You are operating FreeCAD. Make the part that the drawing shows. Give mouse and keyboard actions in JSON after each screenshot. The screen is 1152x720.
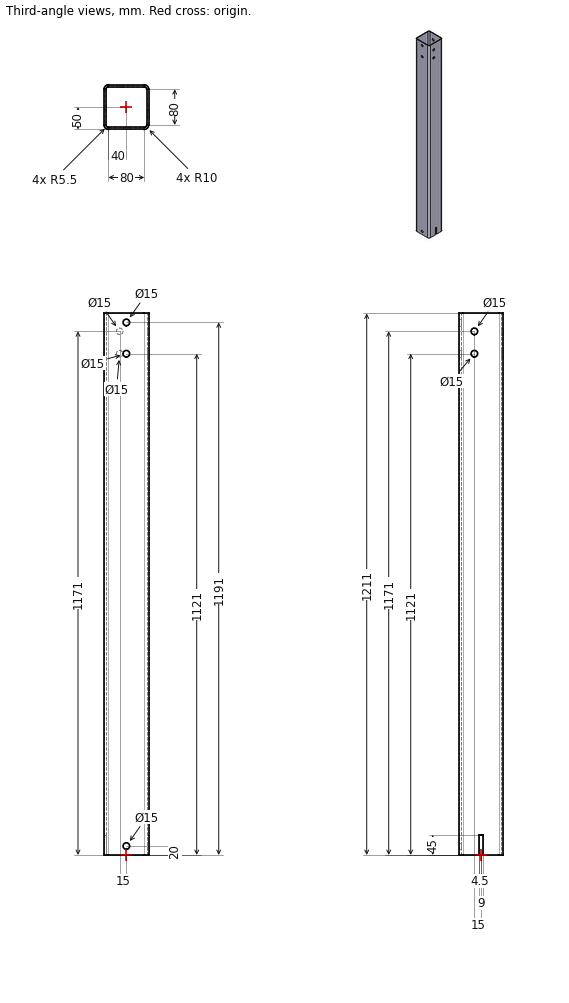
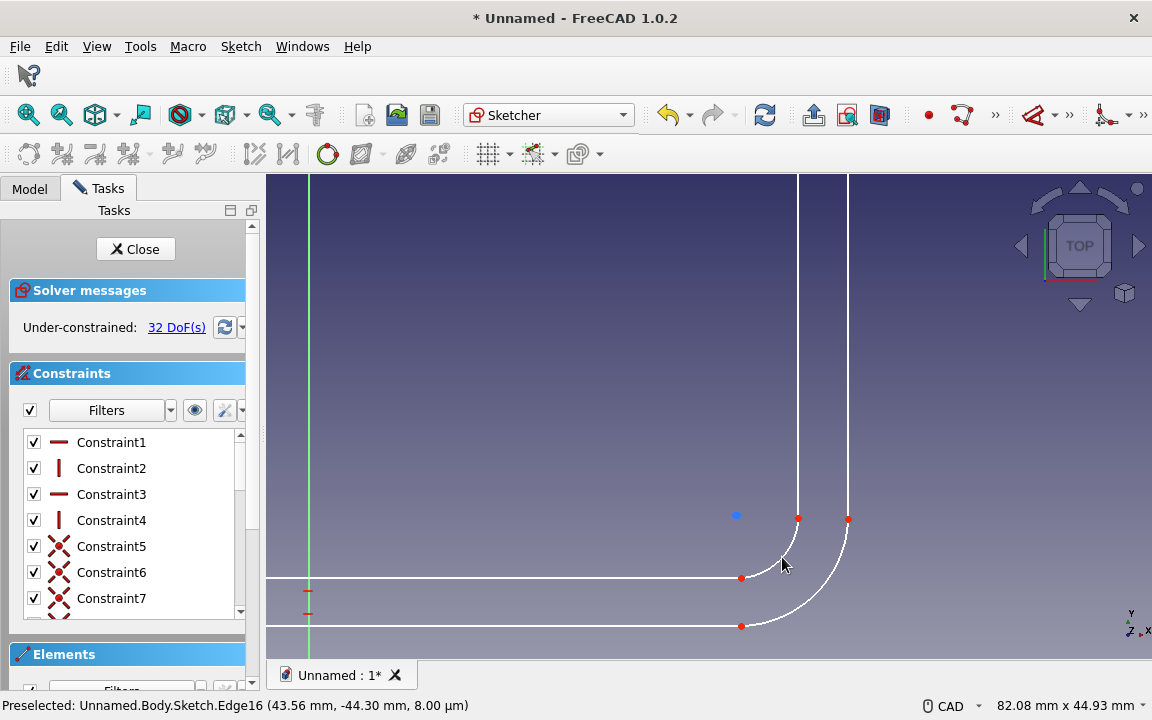
{"action": "left_click", "coordinate": [482, 626]}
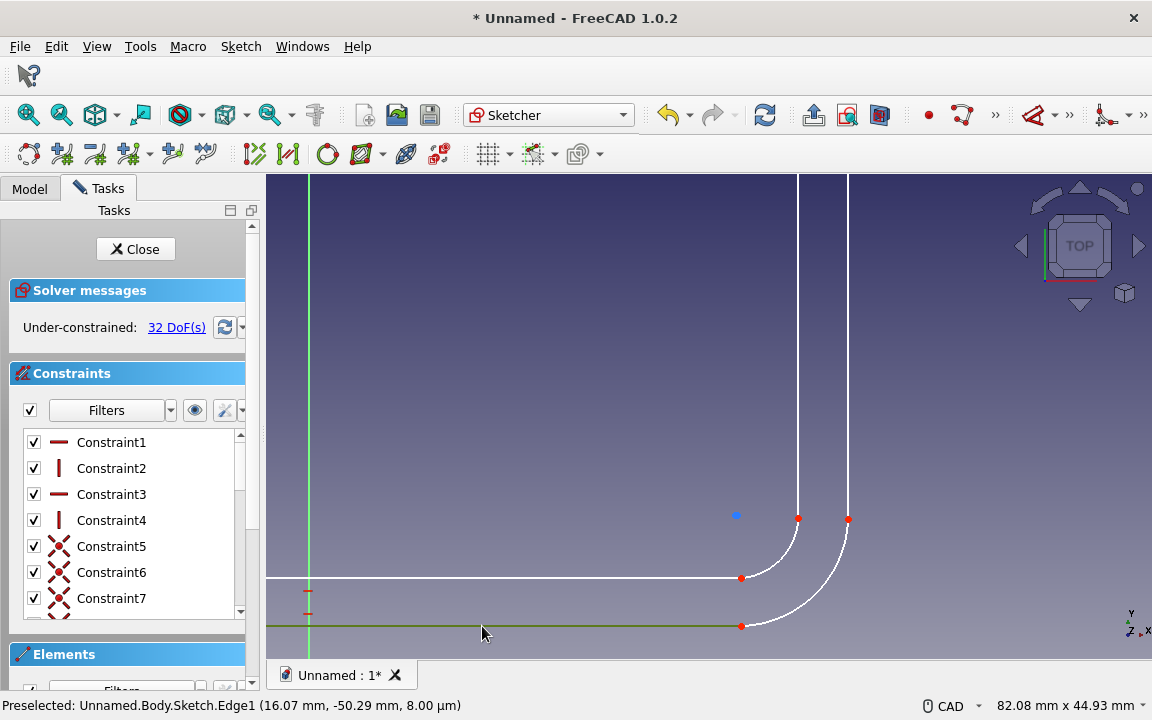
{"action": "left_click", "coordinate": [789, 613]}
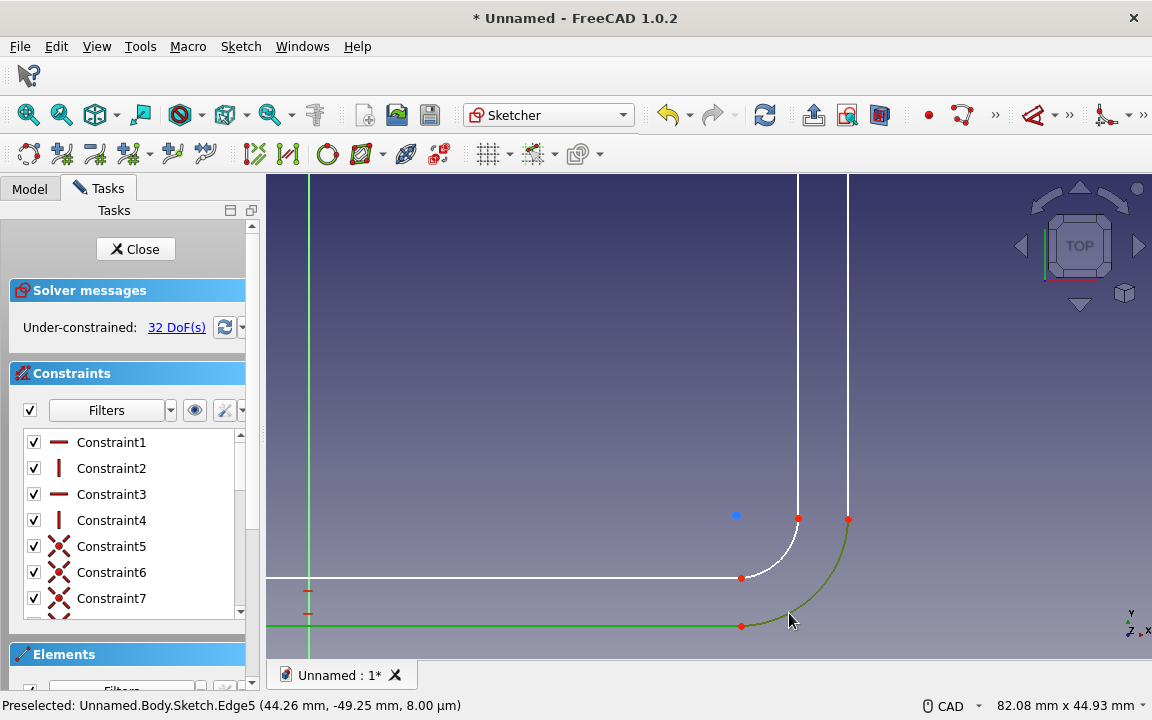
{"action": "key", "text": "t"}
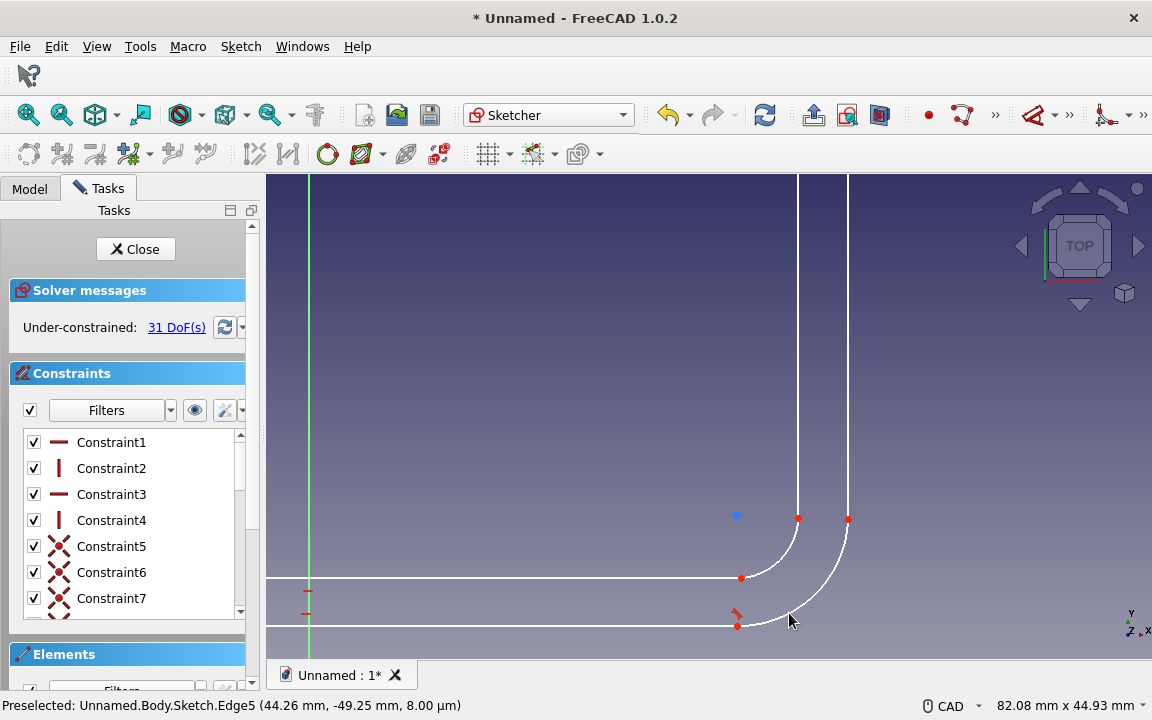
{"action": "left_click", "coordinate": [479, 626]}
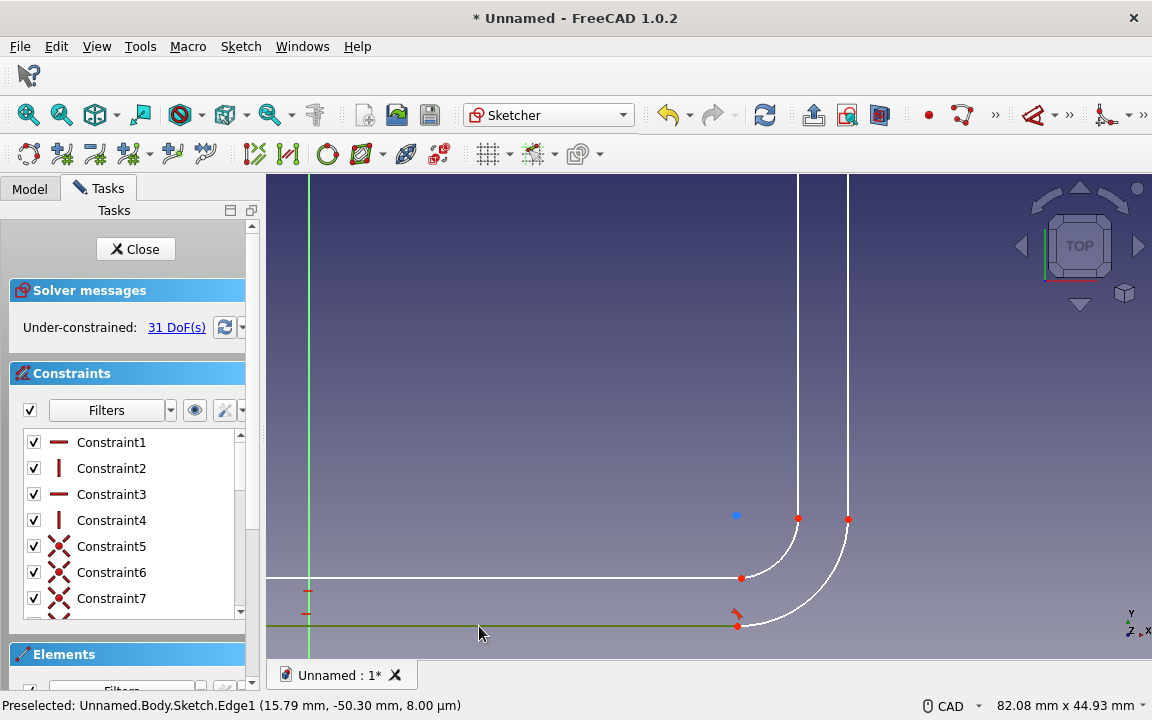
{"action": "scroll", "coordinate": [784, 560], "scroll_direction": "down", "scroll_amount": 6}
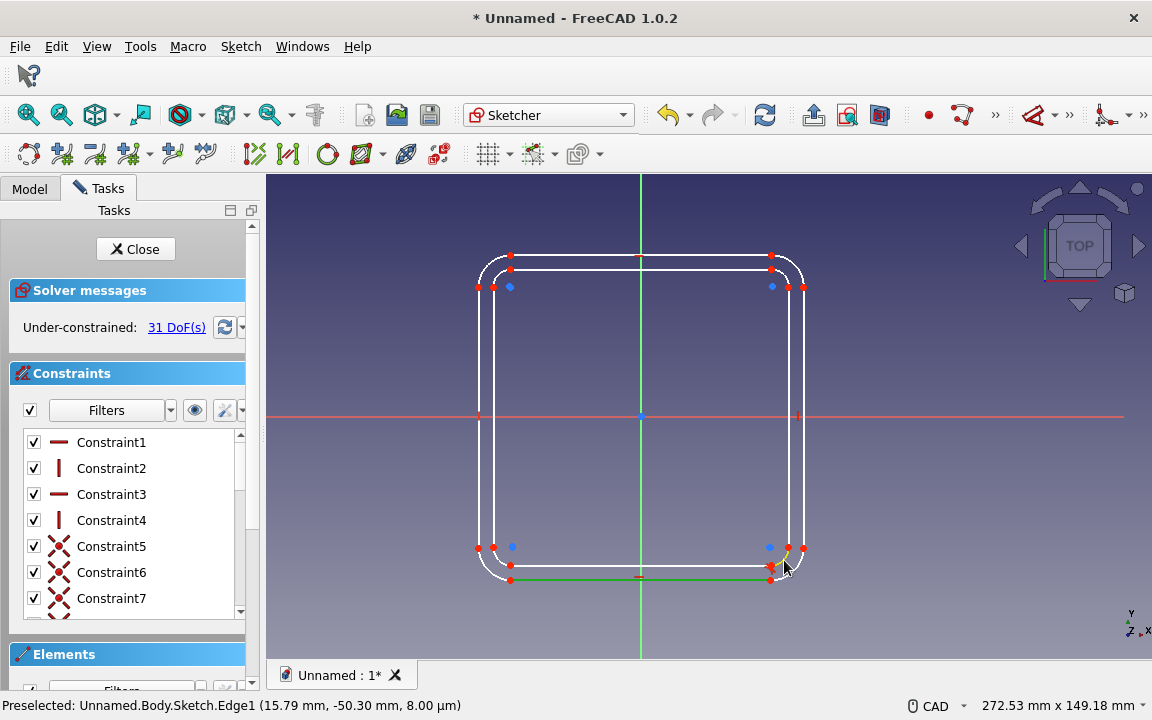
{"action": "left_click", "coordinate": [483, 563]}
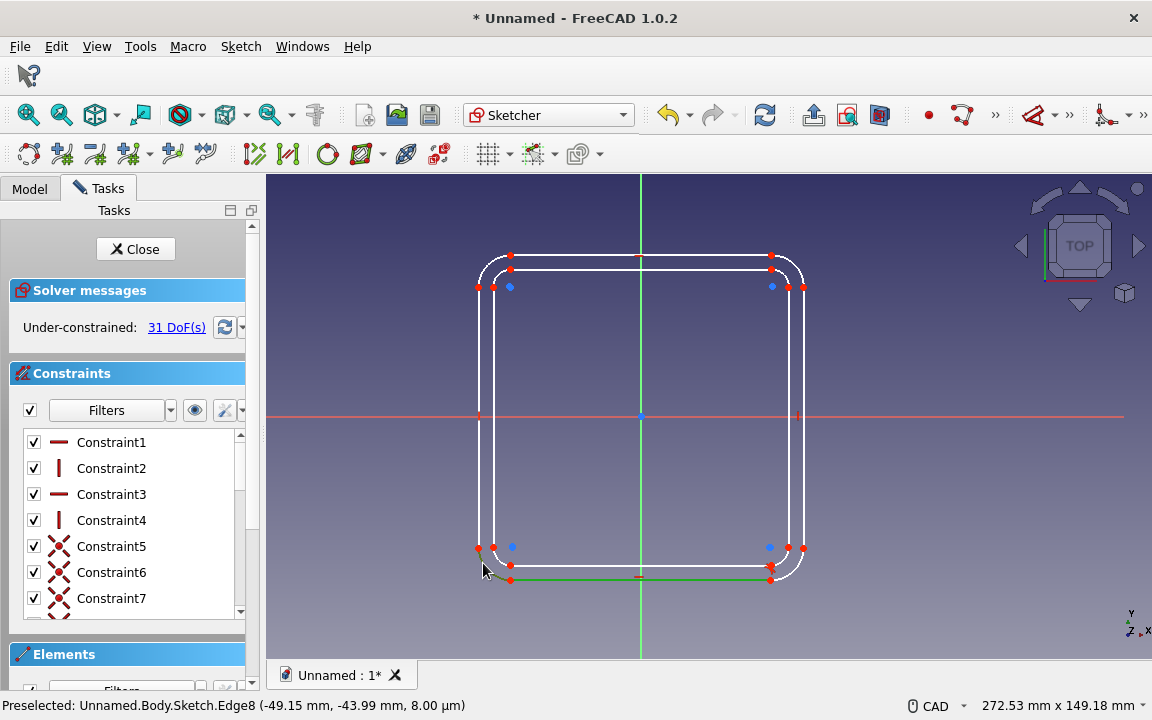
{"action": "key", "text": "t"}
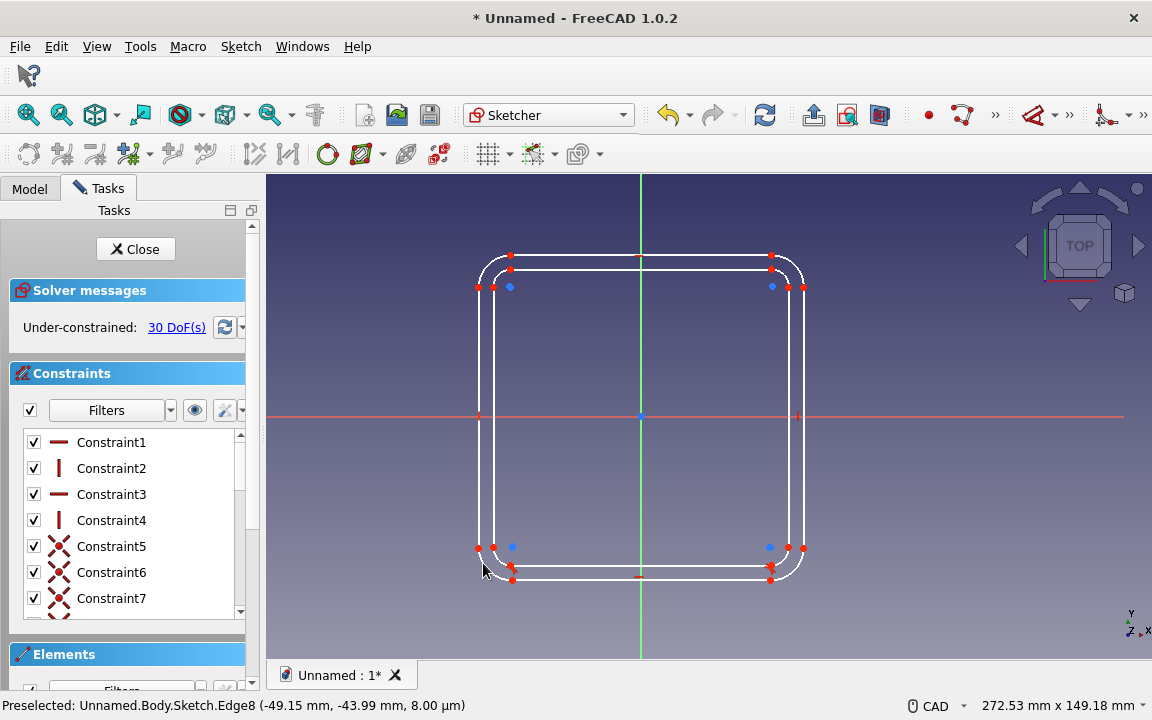
{"action": "left_click", "coordinate": [804, 470]}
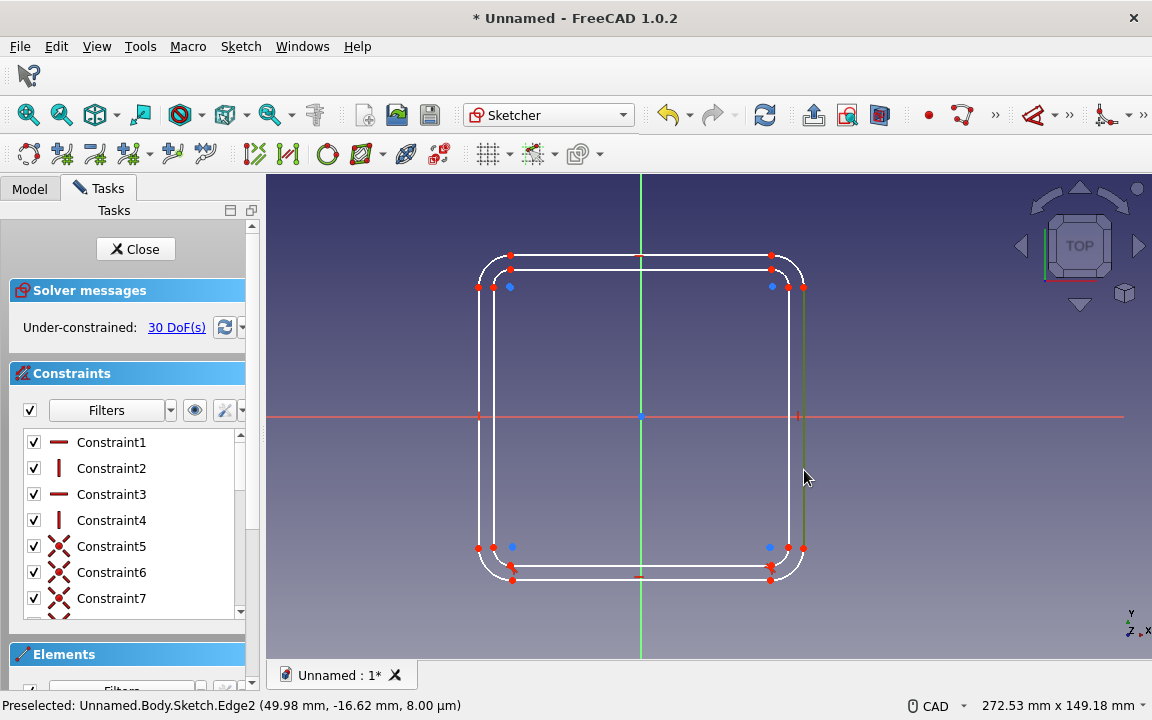
{"action": "left_click", "coordinate": [785, 577]}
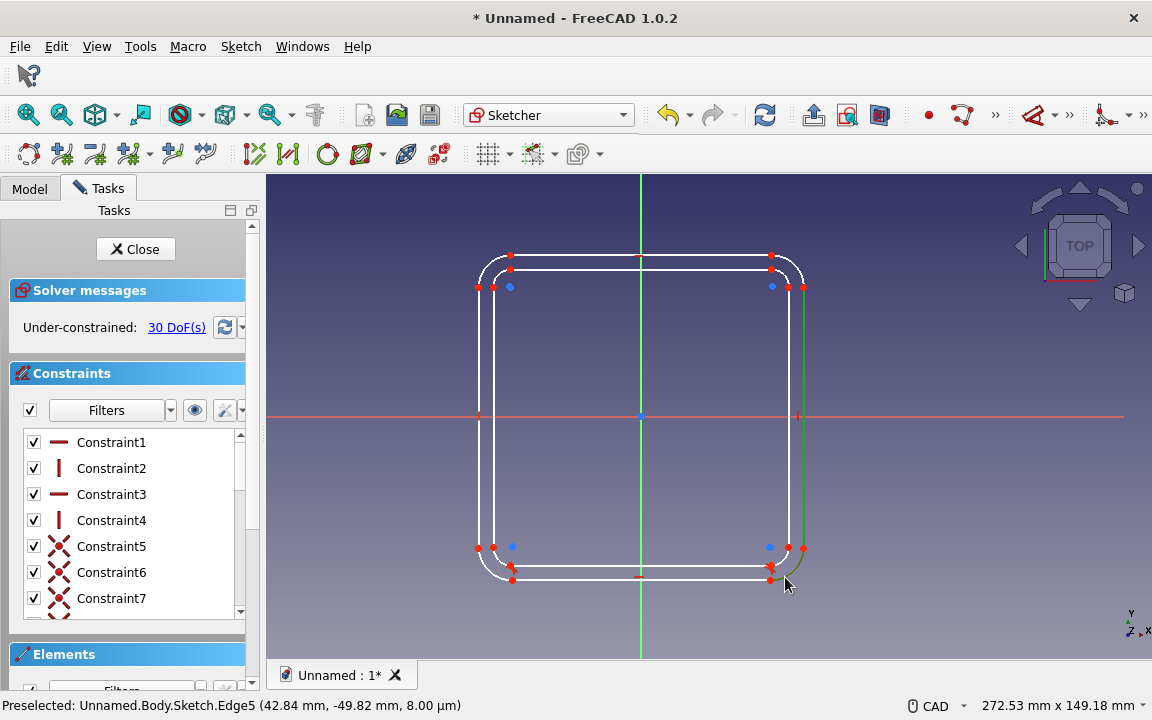
{"action": "key", "text": "t"}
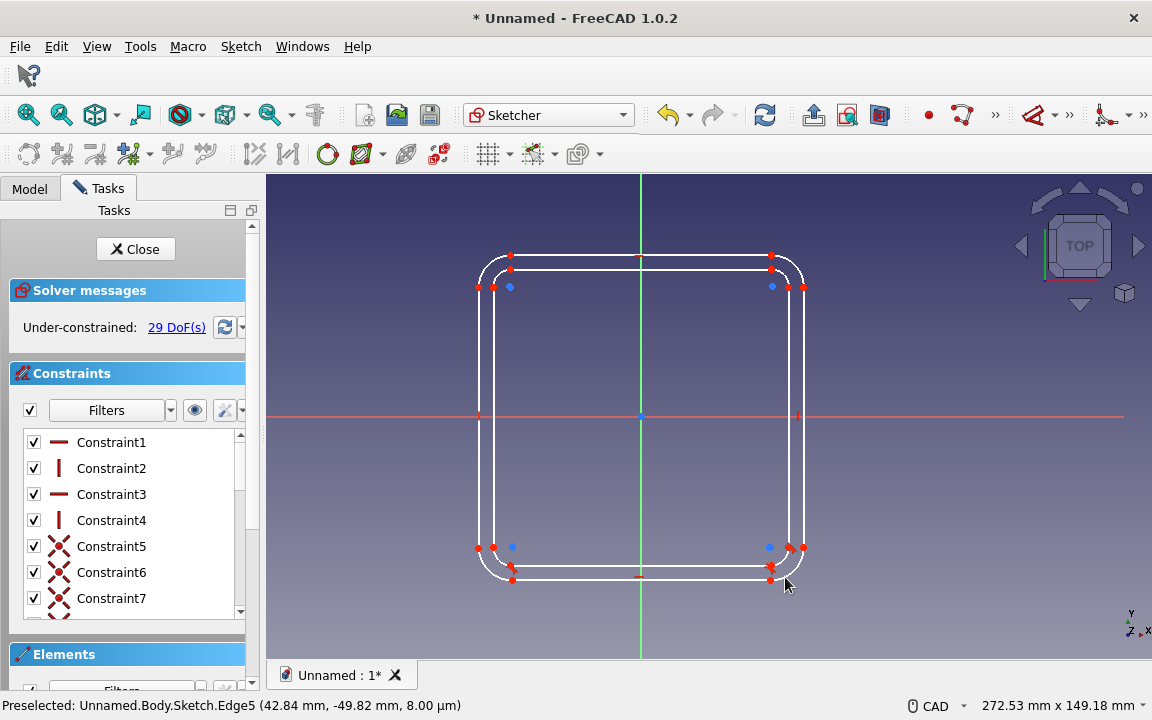
{"action": "left_click", "coordinate": [804, 469]}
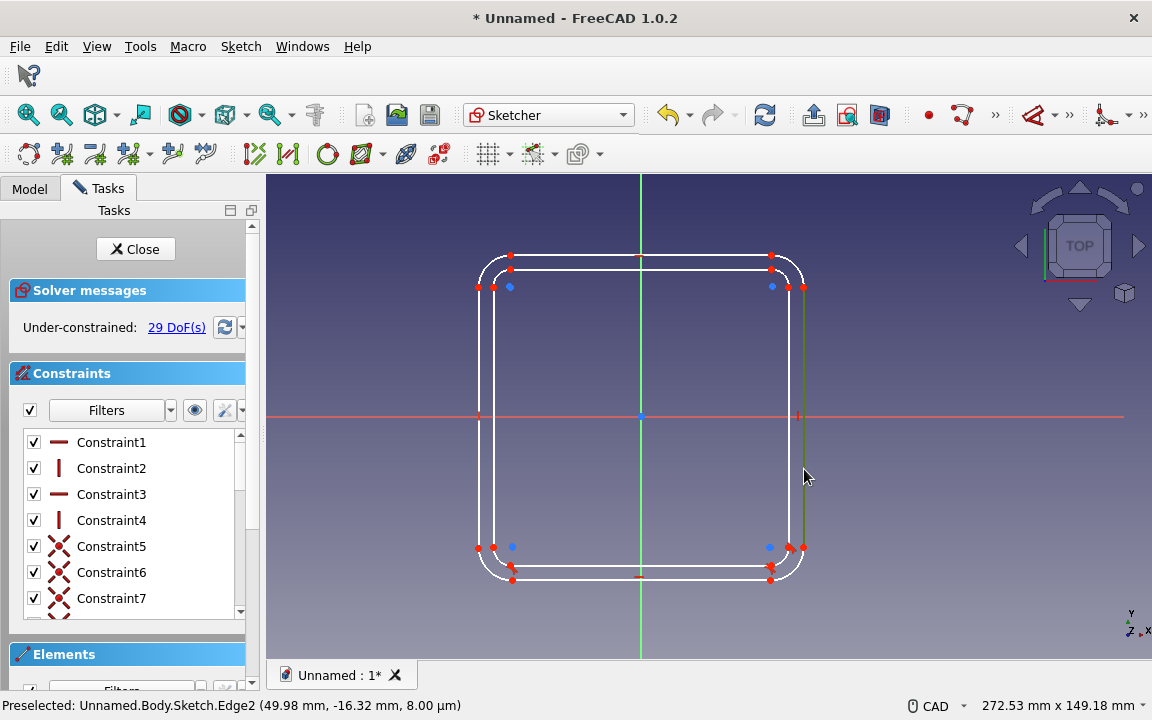
{"action": "left_click", "coordinate": [800, 273]}